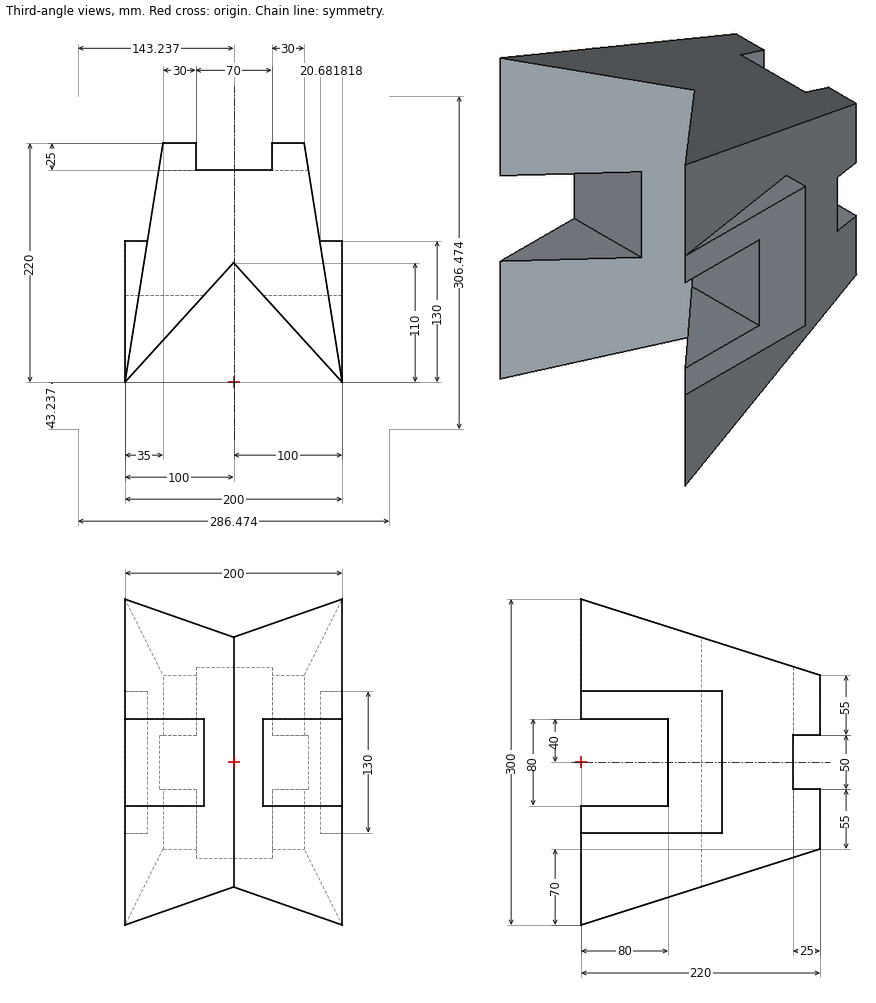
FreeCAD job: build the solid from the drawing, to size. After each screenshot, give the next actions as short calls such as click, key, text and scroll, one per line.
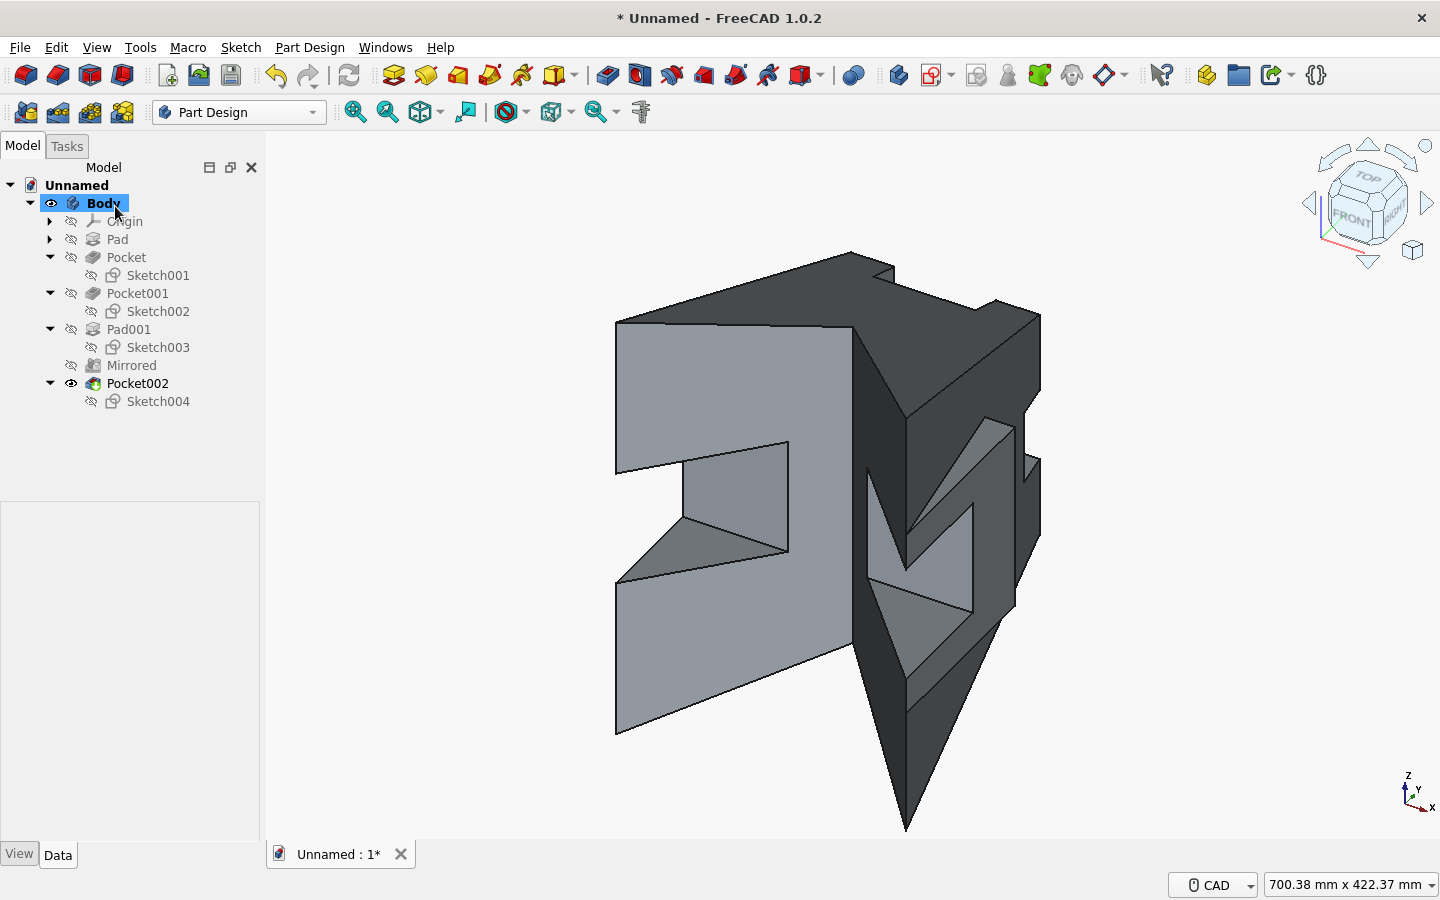
key(0)